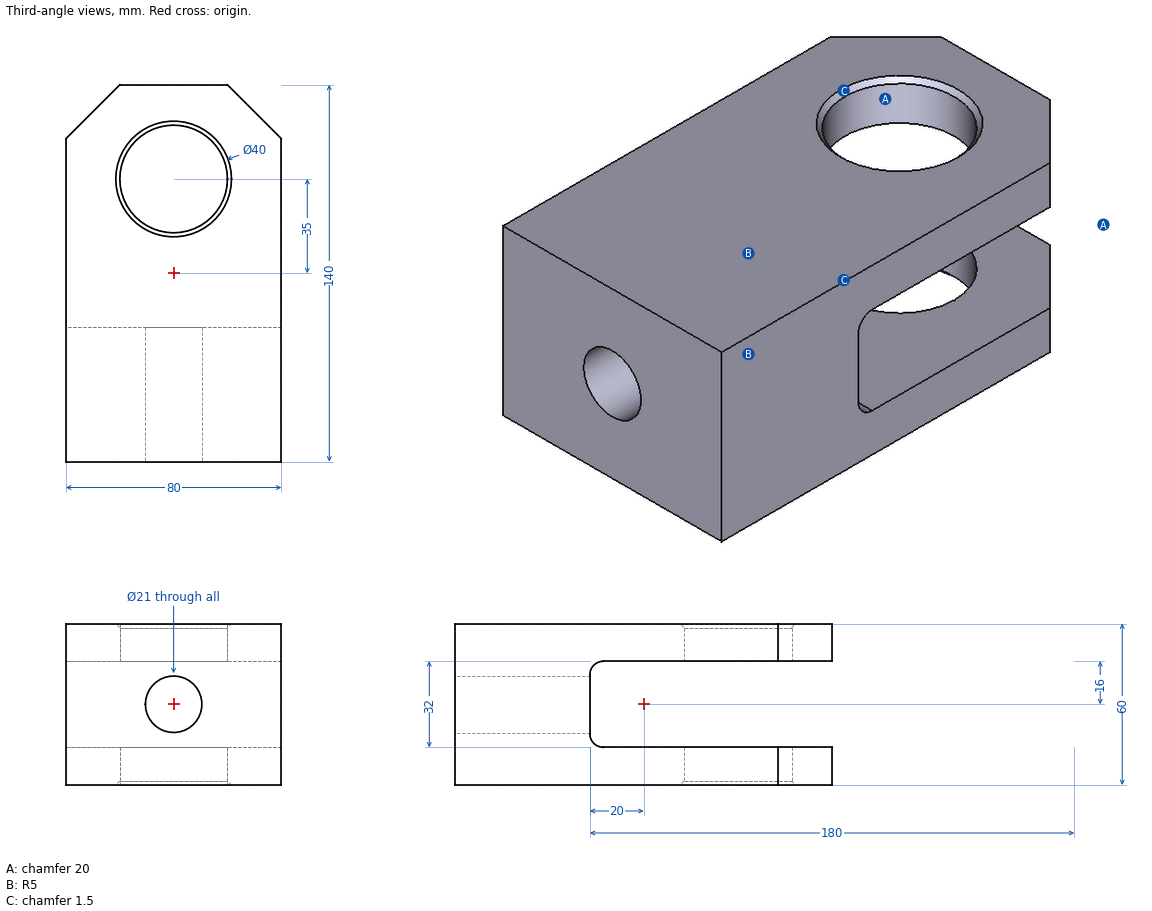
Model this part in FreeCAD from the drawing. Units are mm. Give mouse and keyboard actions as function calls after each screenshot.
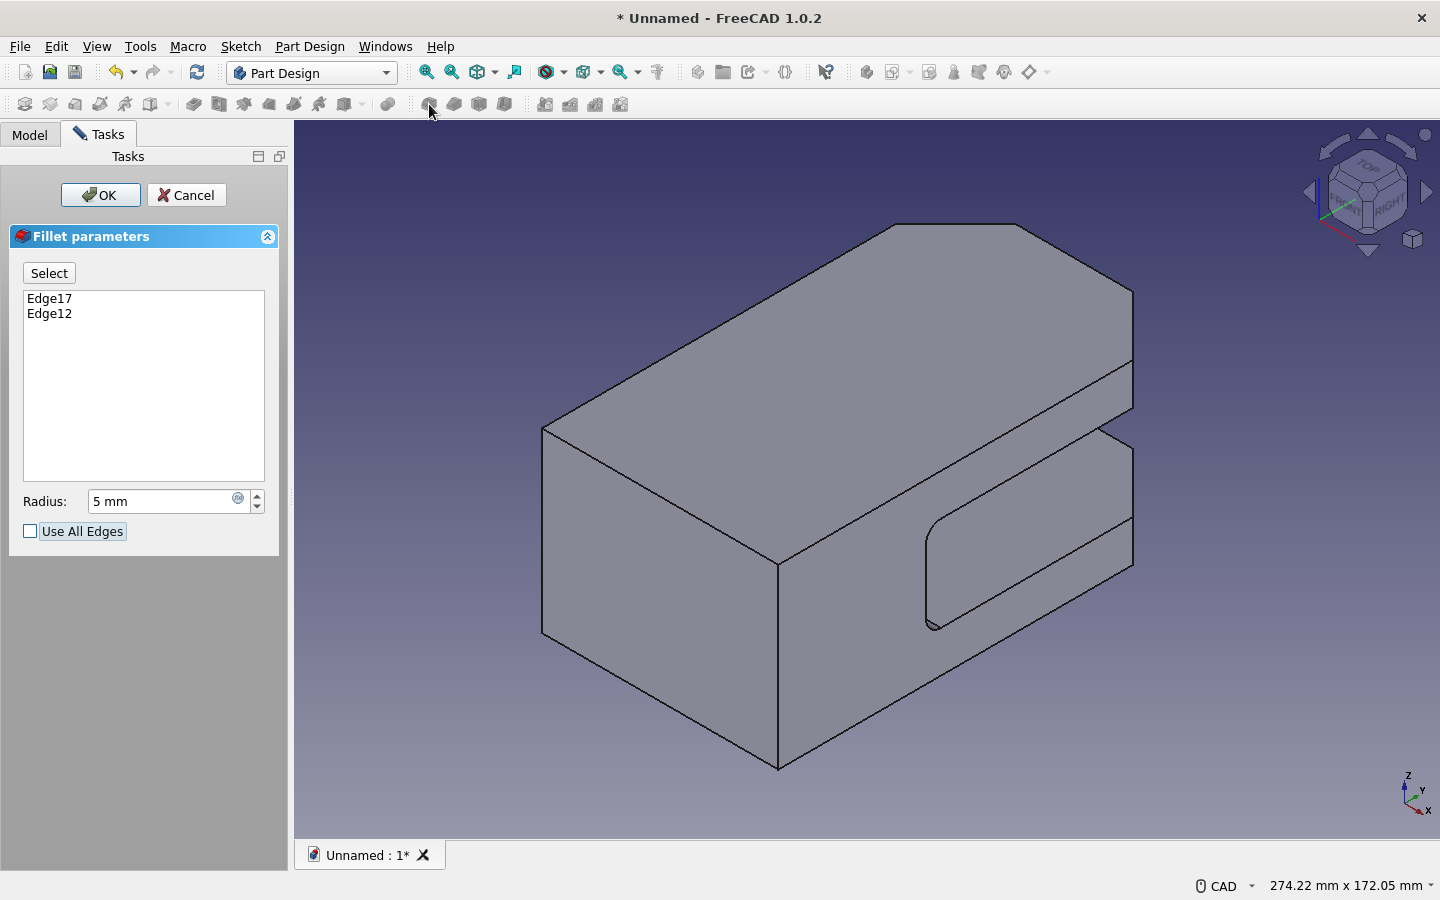
click(101, 195)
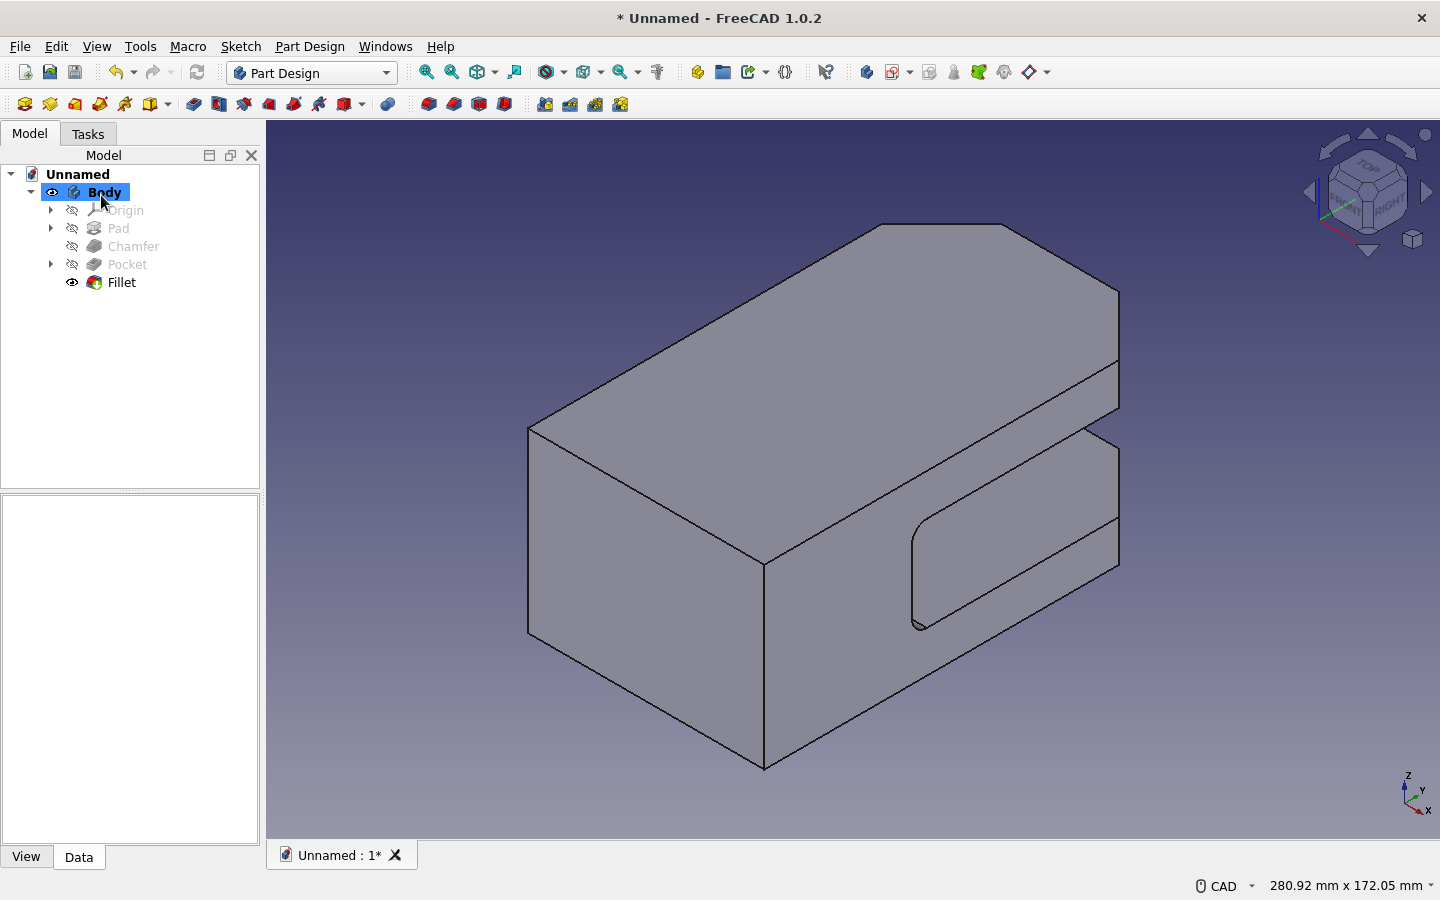
click(912, 342)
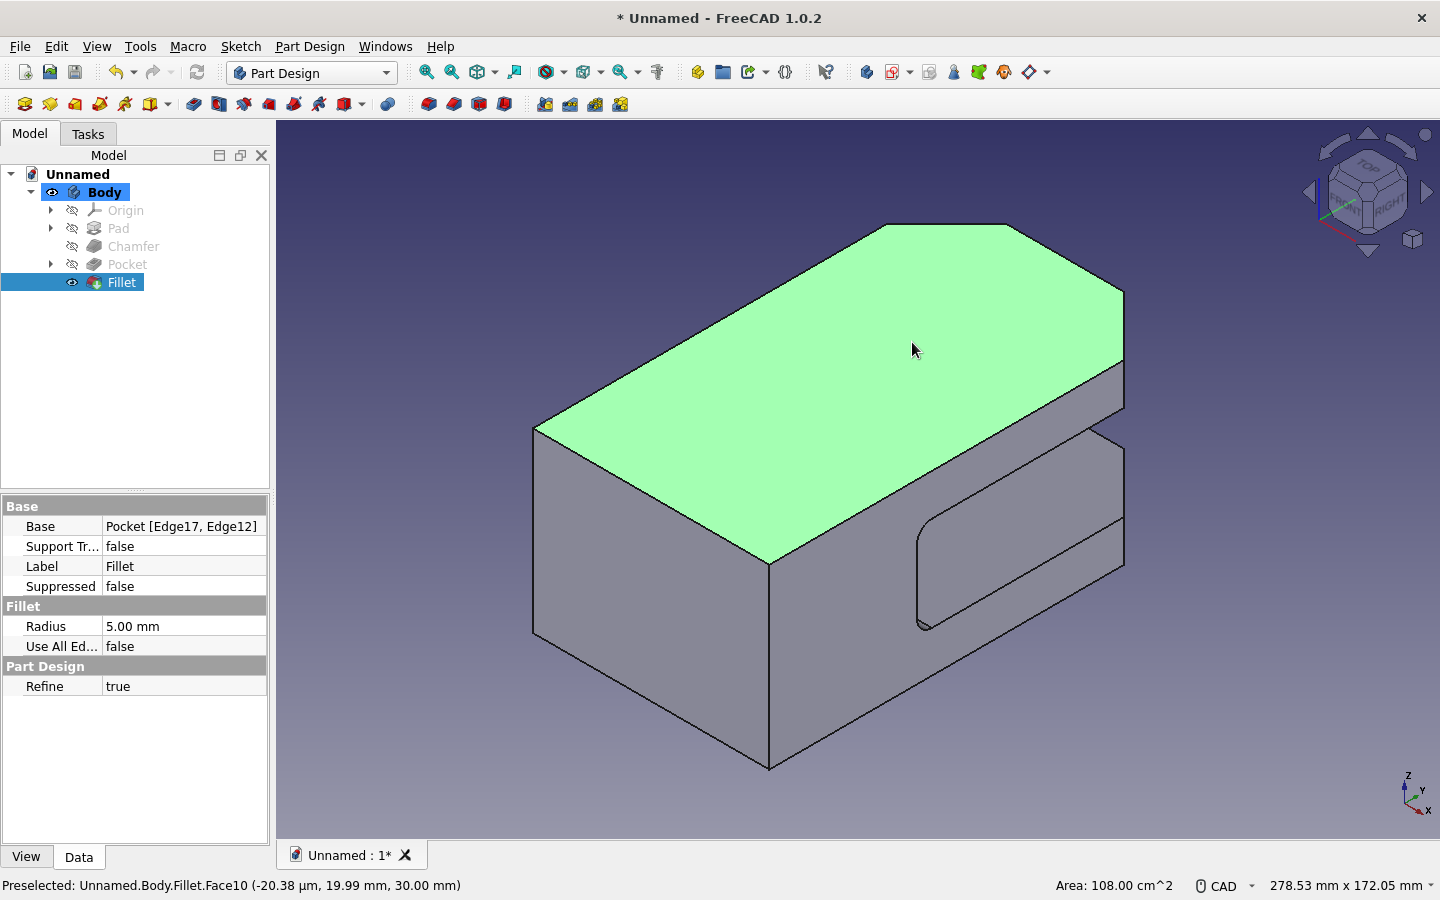
click(892, 72)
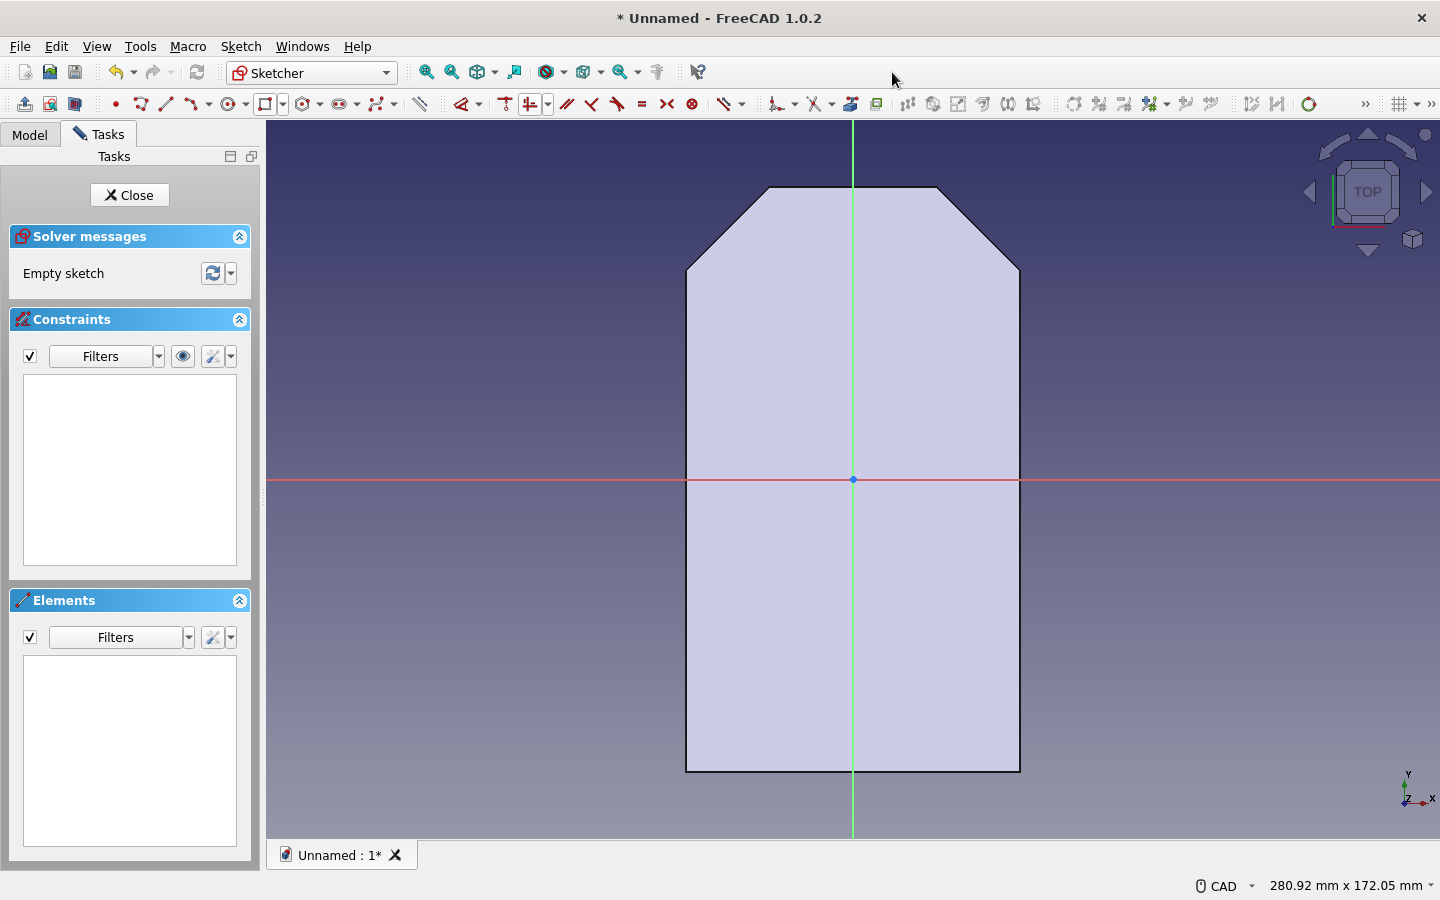
scroll(909, 271, up, 4)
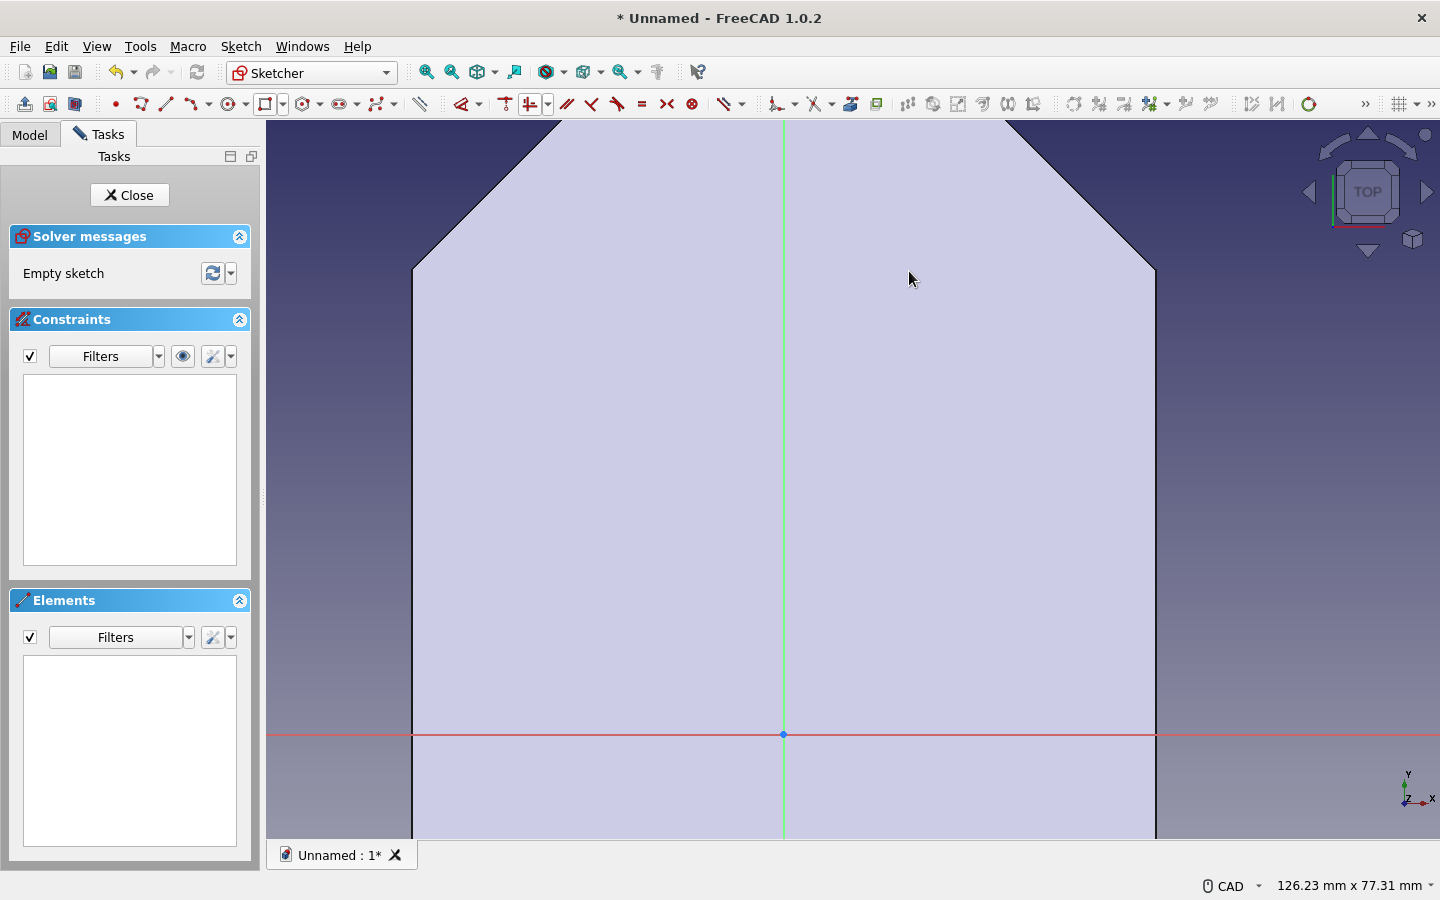
click(228, 104)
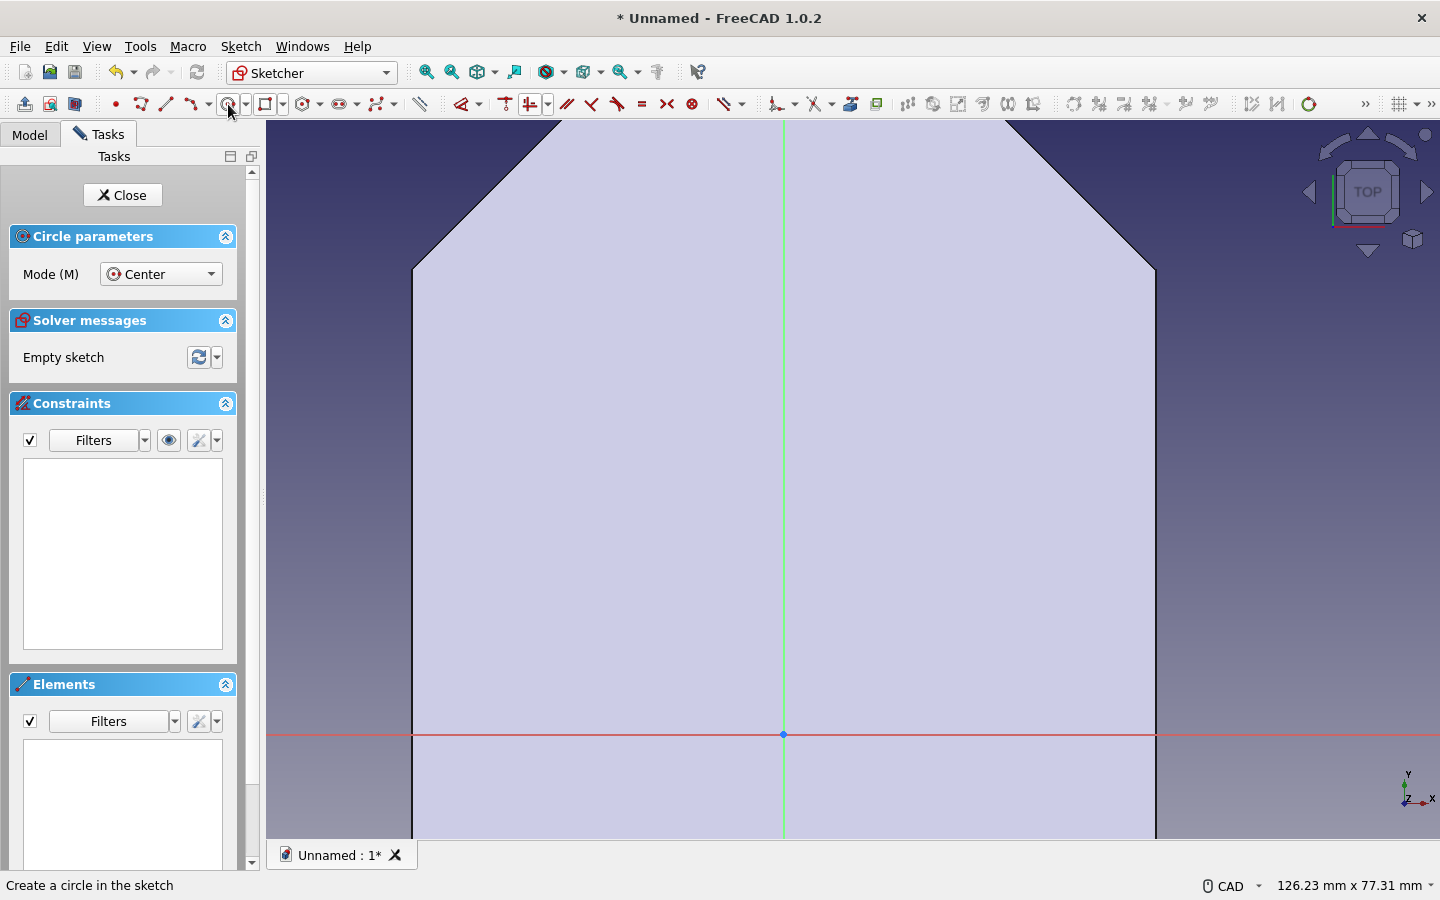
click(784, 409)
move(915, 278)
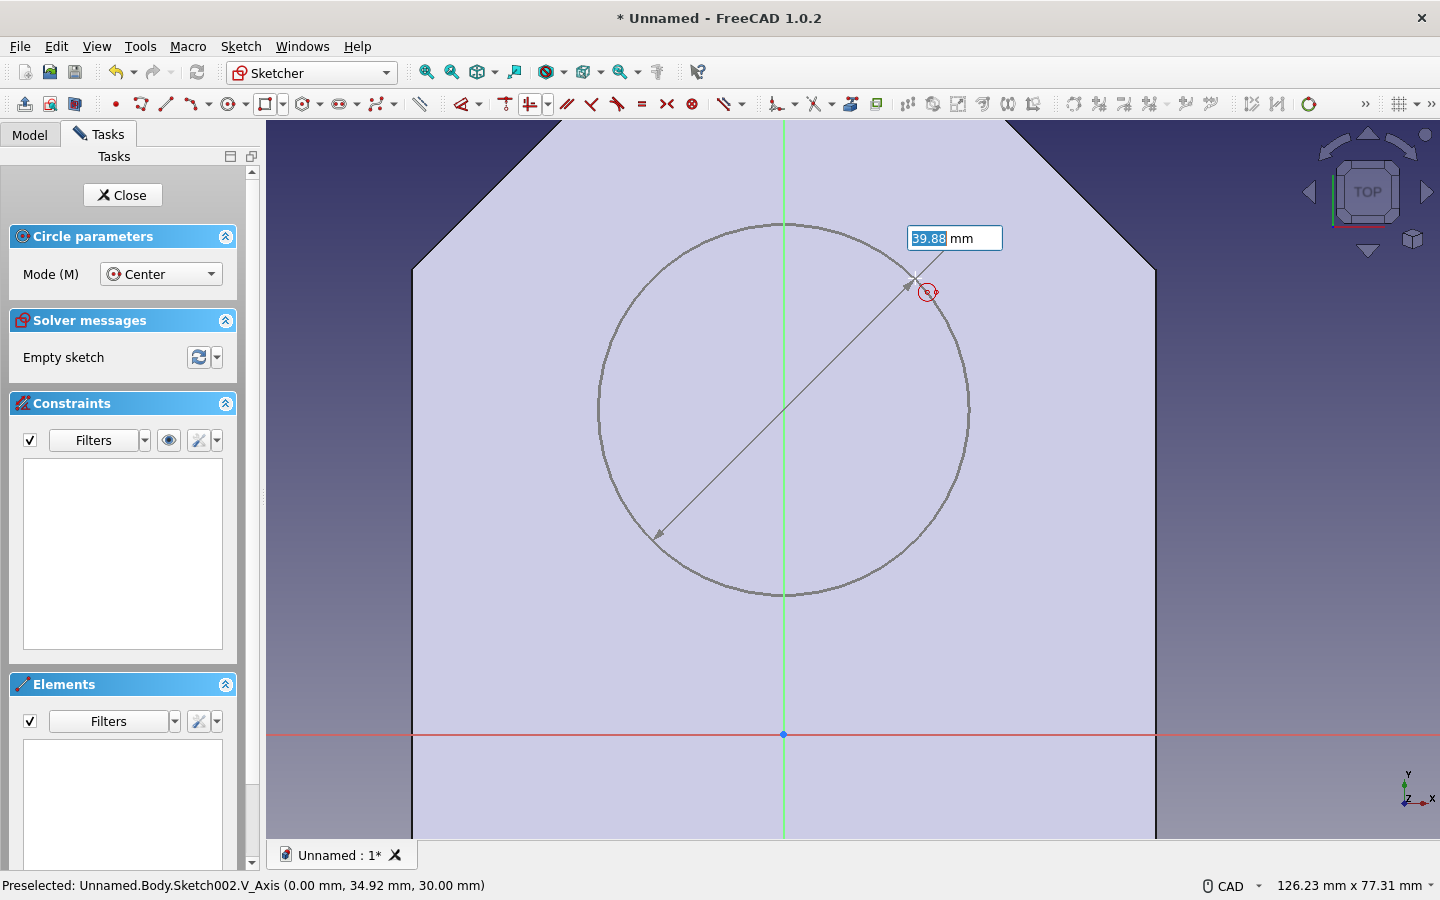
text(40)
key(Return)
key(Escape)